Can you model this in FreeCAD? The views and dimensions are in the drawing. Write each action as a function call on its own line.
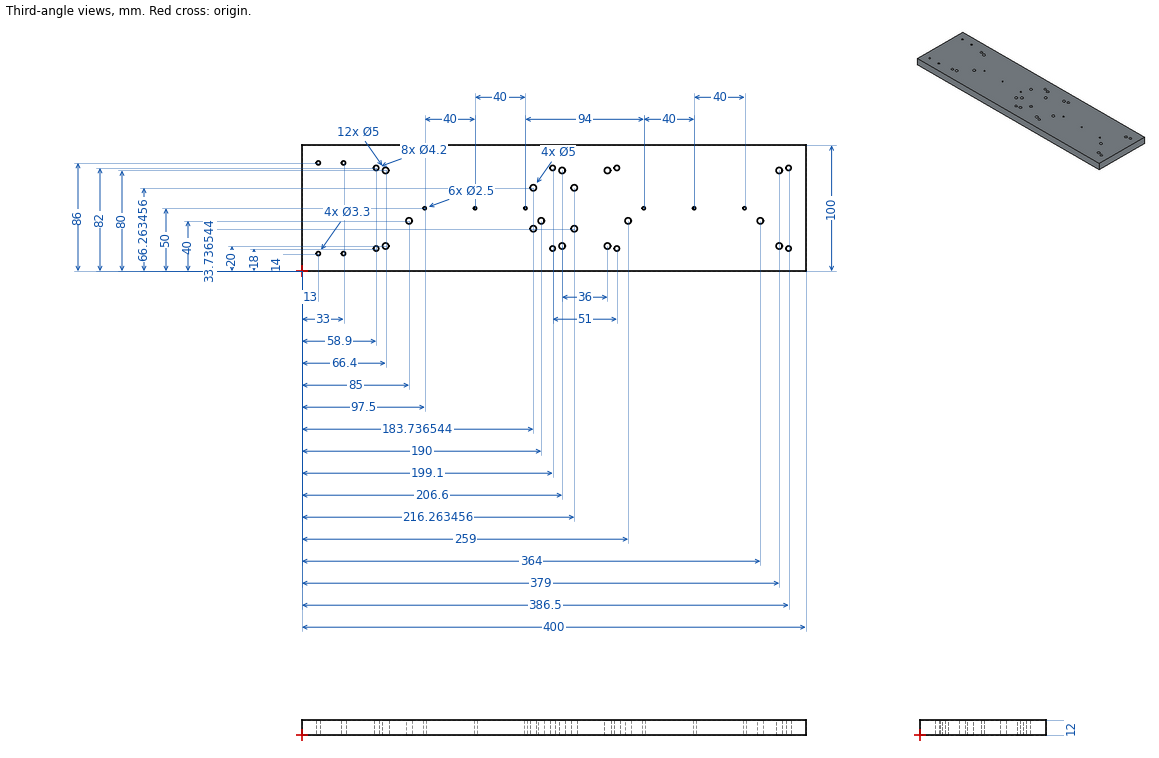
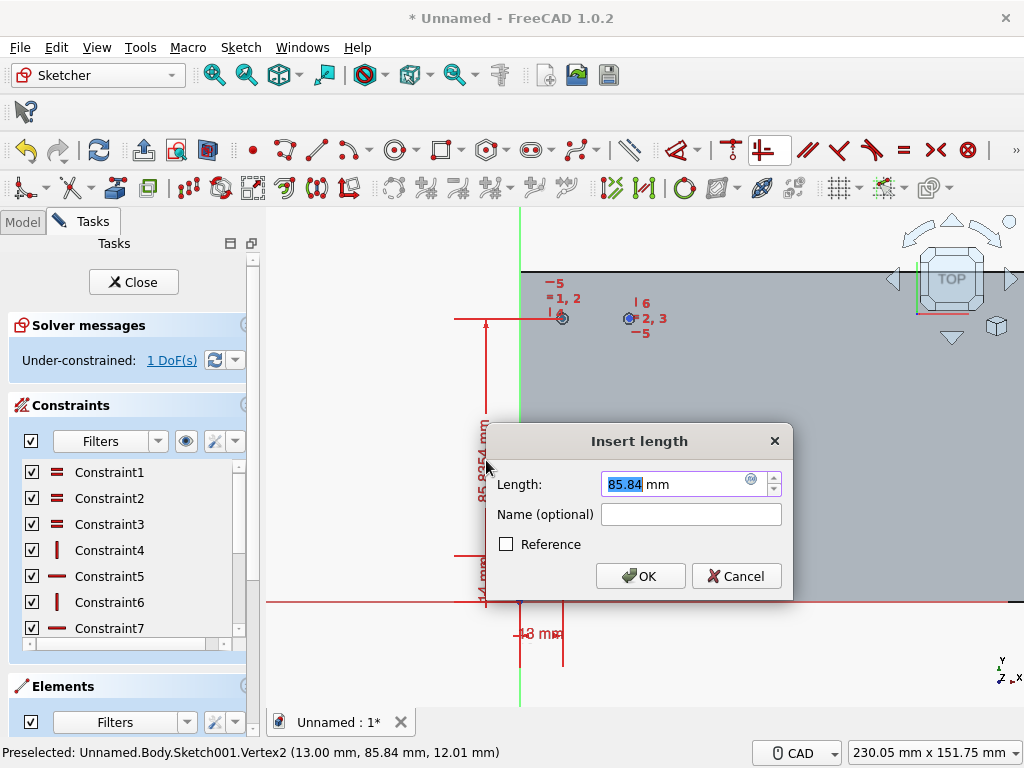
text(86)
key(Return)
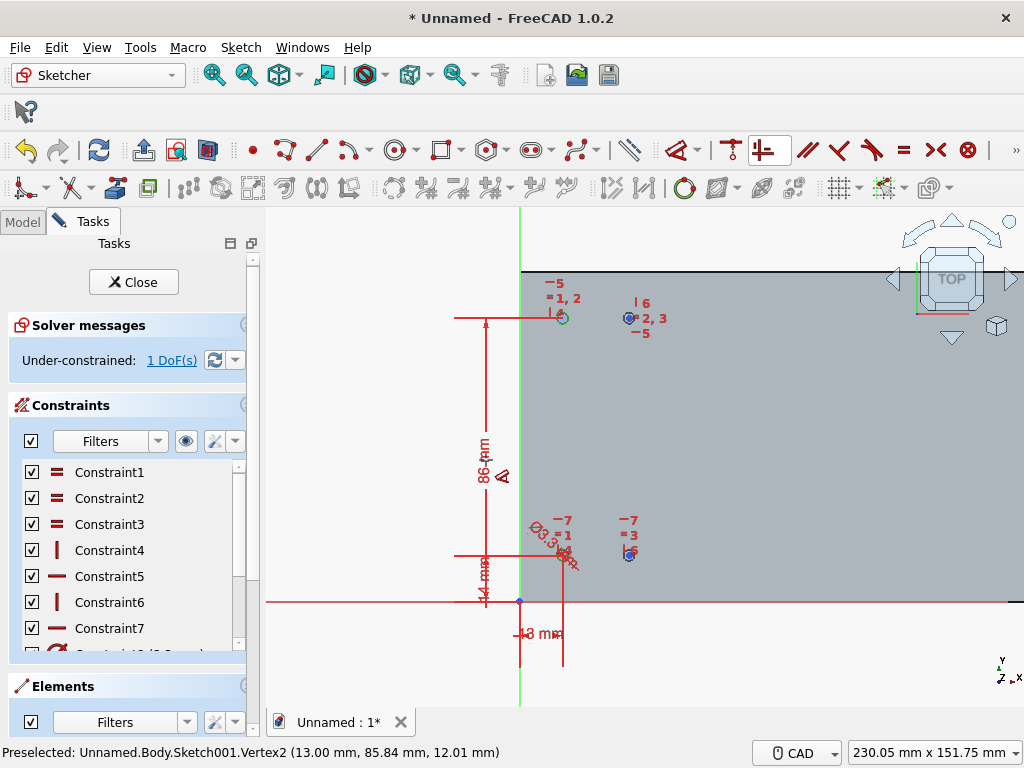
click(629, 318)
click(613, 636)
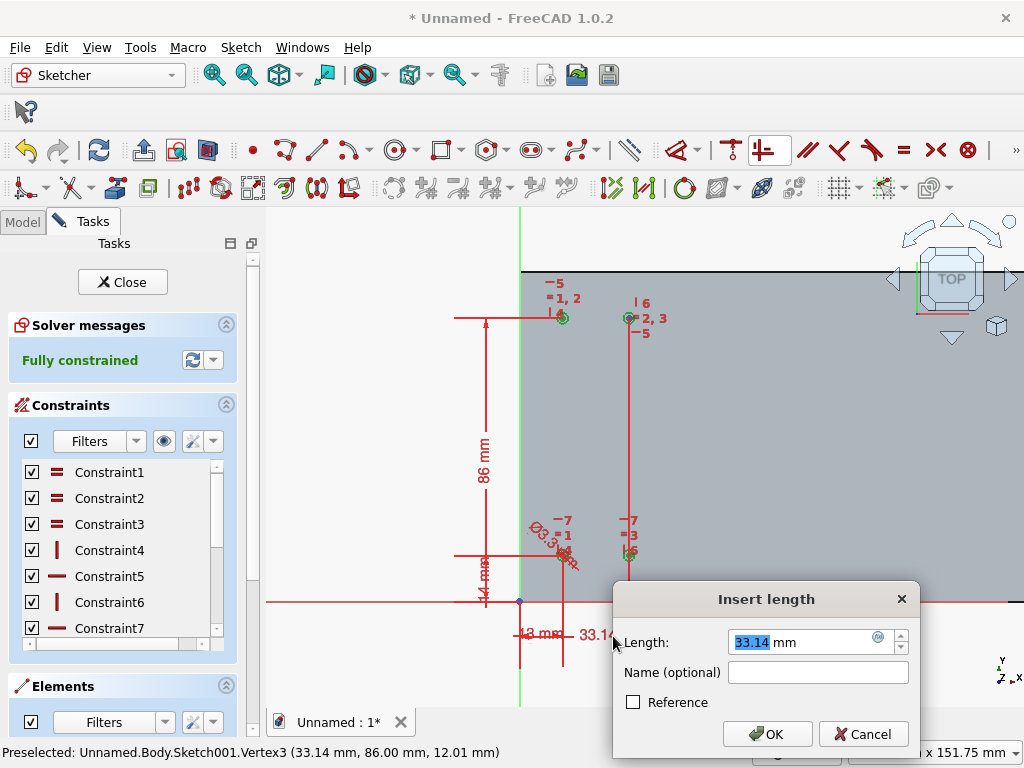
text(33)
key(Return)
key(Escape)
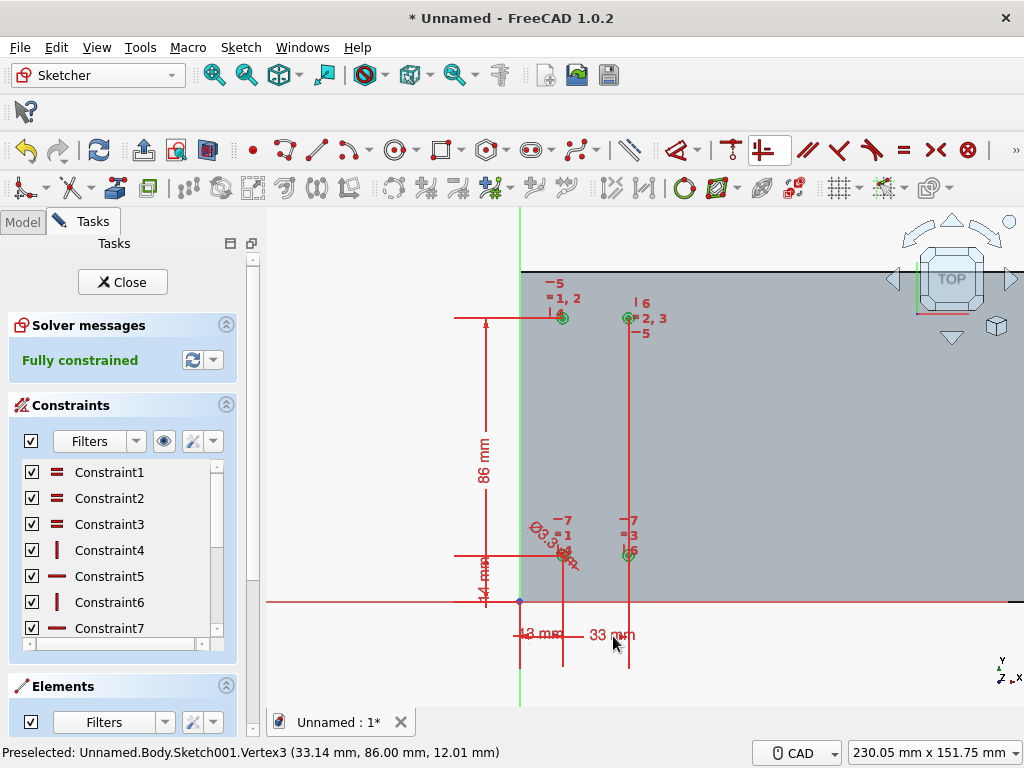
click(123, 282)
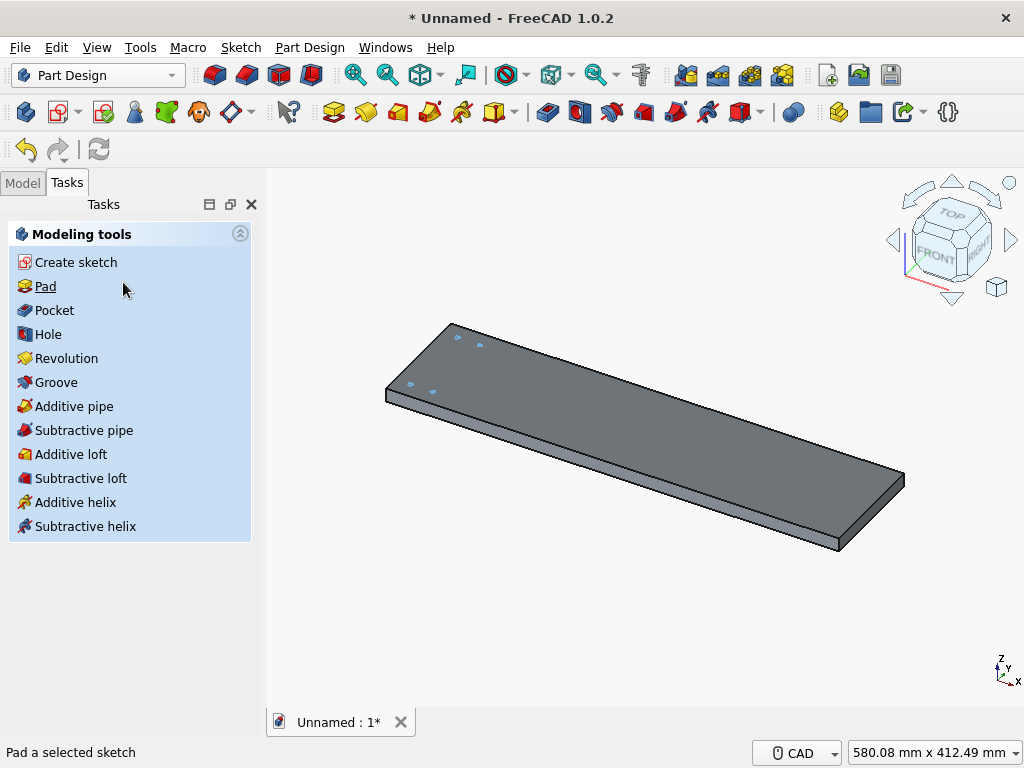
click(548, 112)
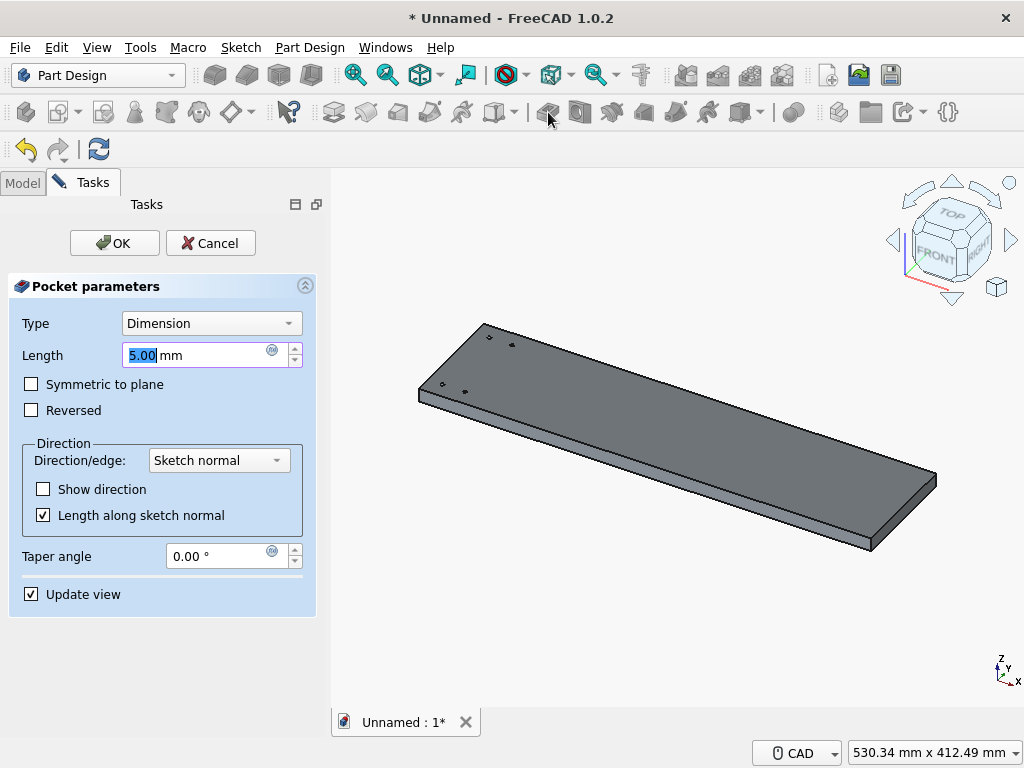
click(212, 324)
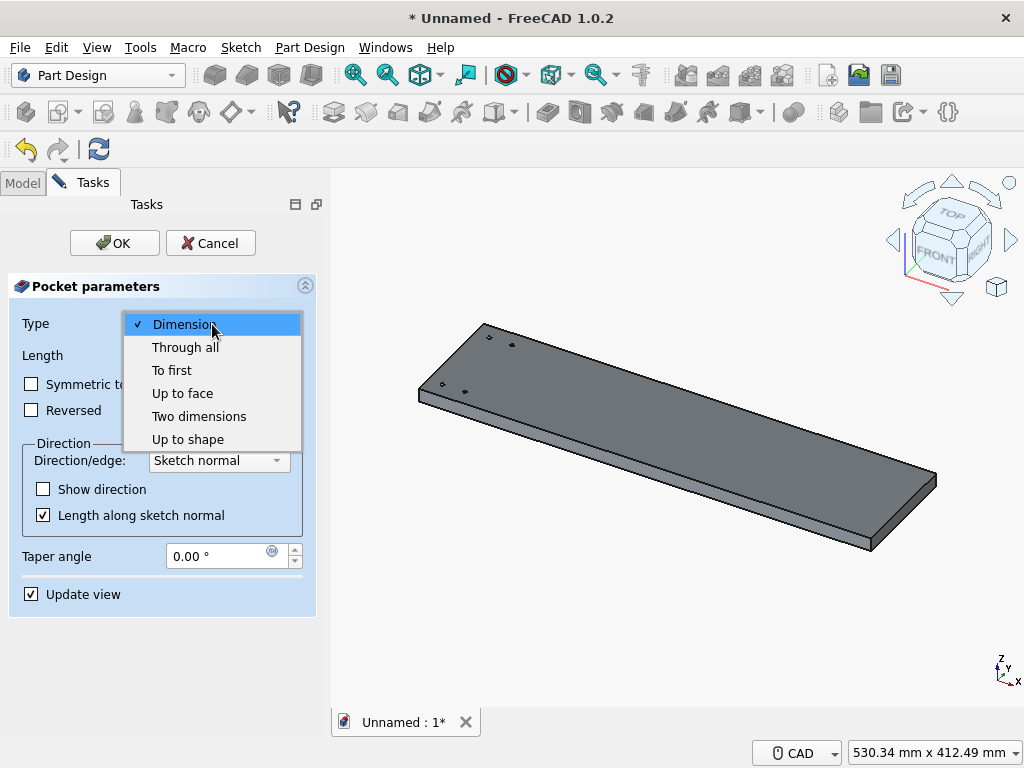
click(212, 348)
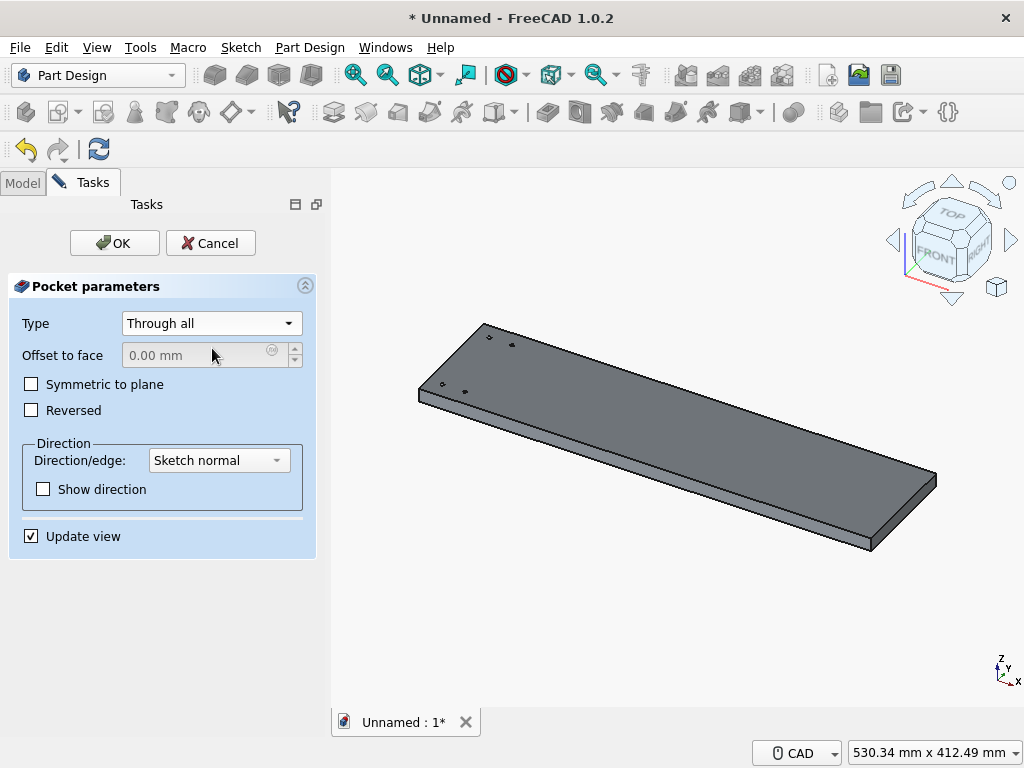
click(115, 243)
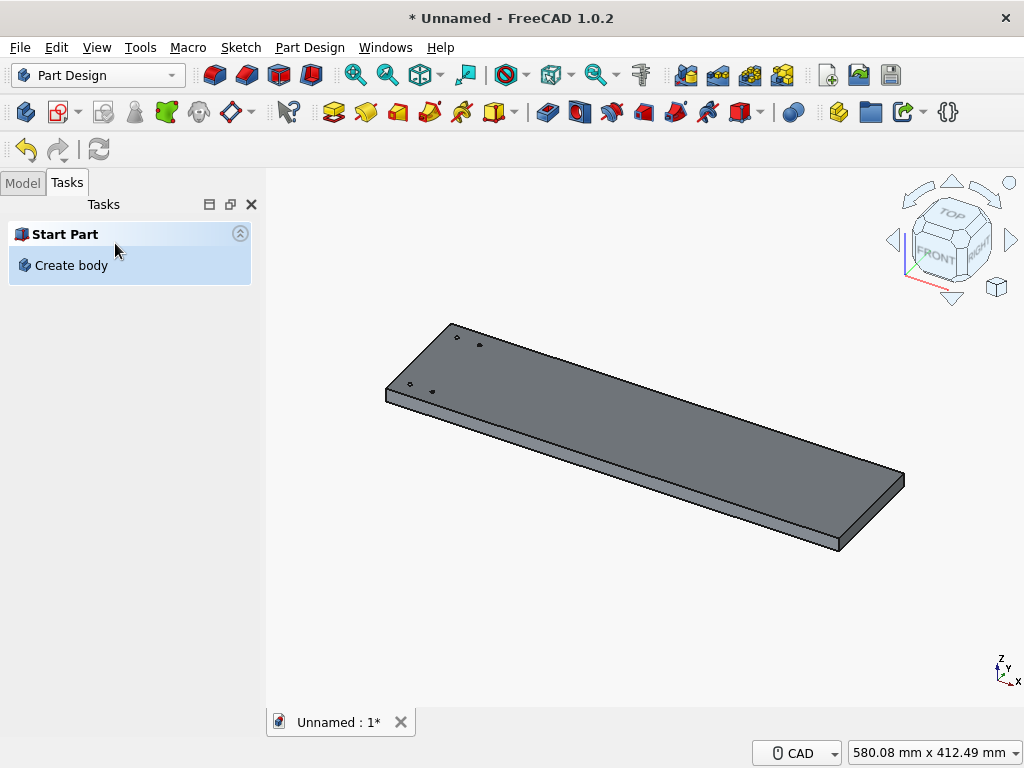
click(774, 473)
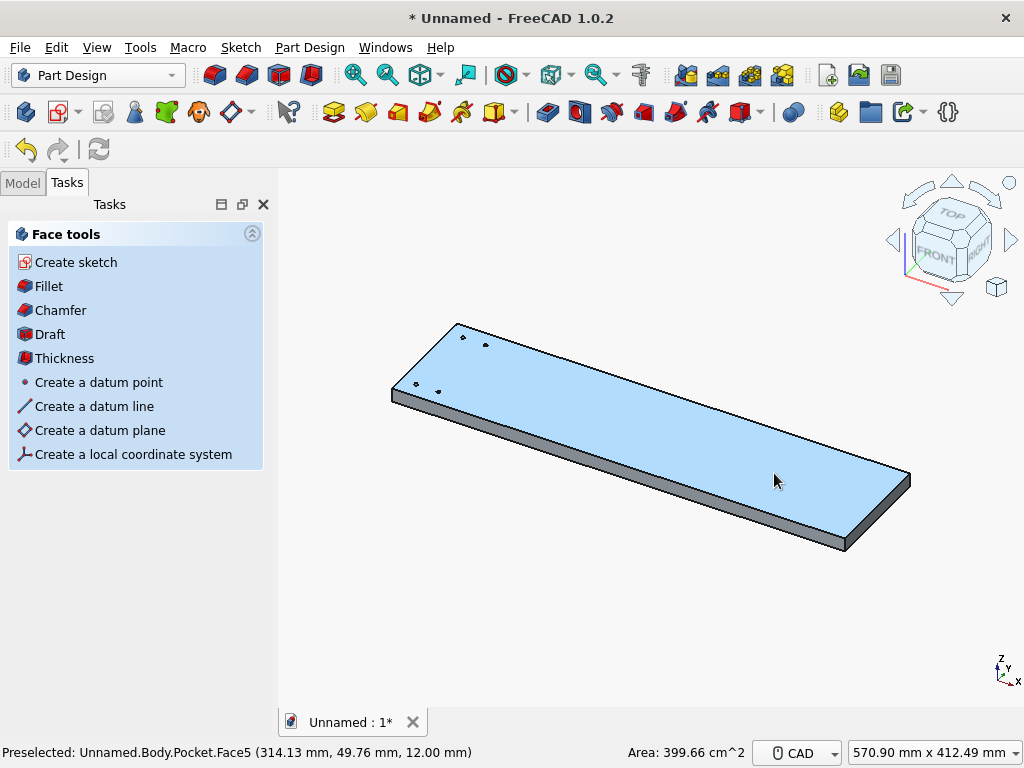
click(58, 112)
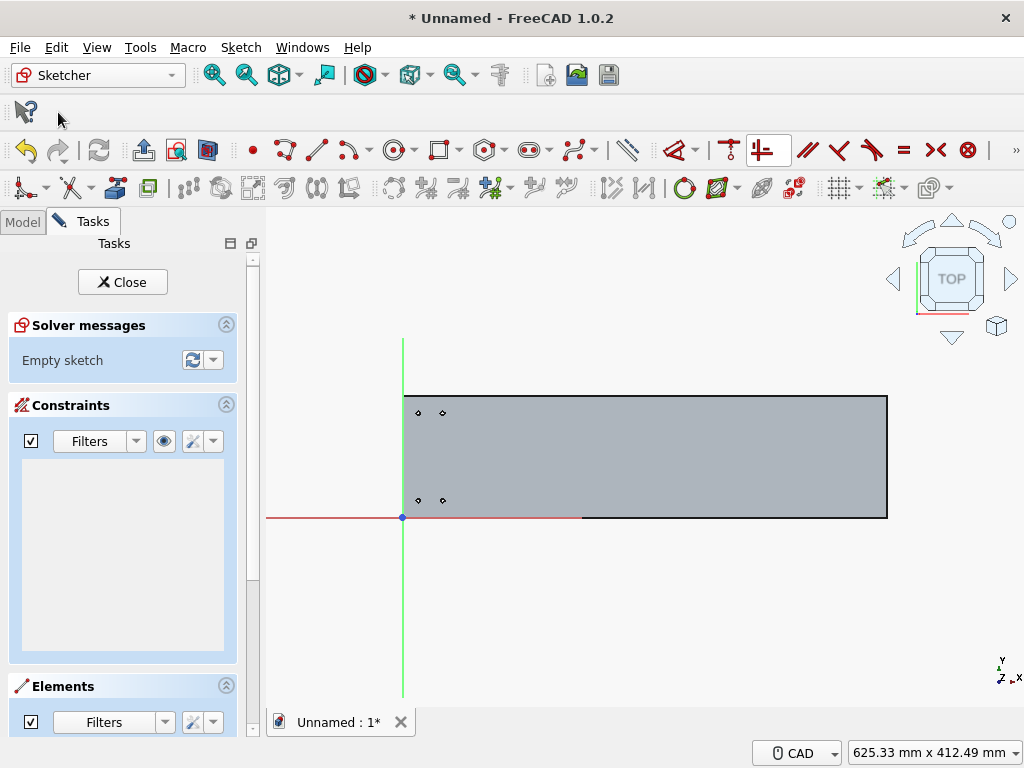
scroll(298, 413, down, 1)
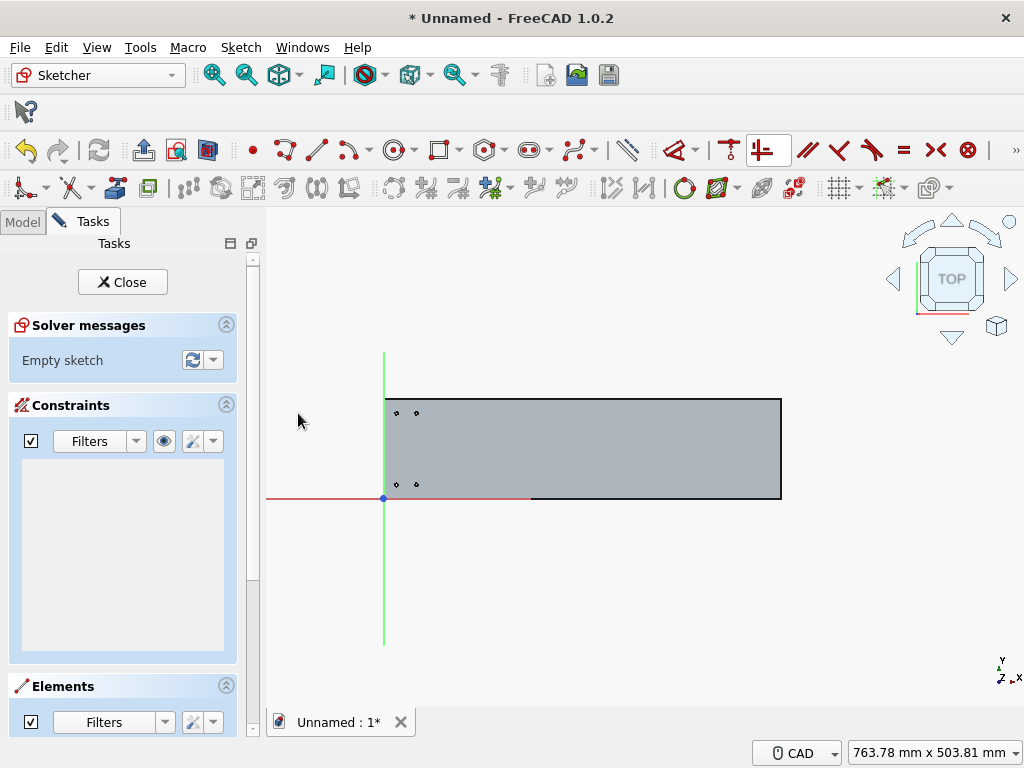
click(394, 150)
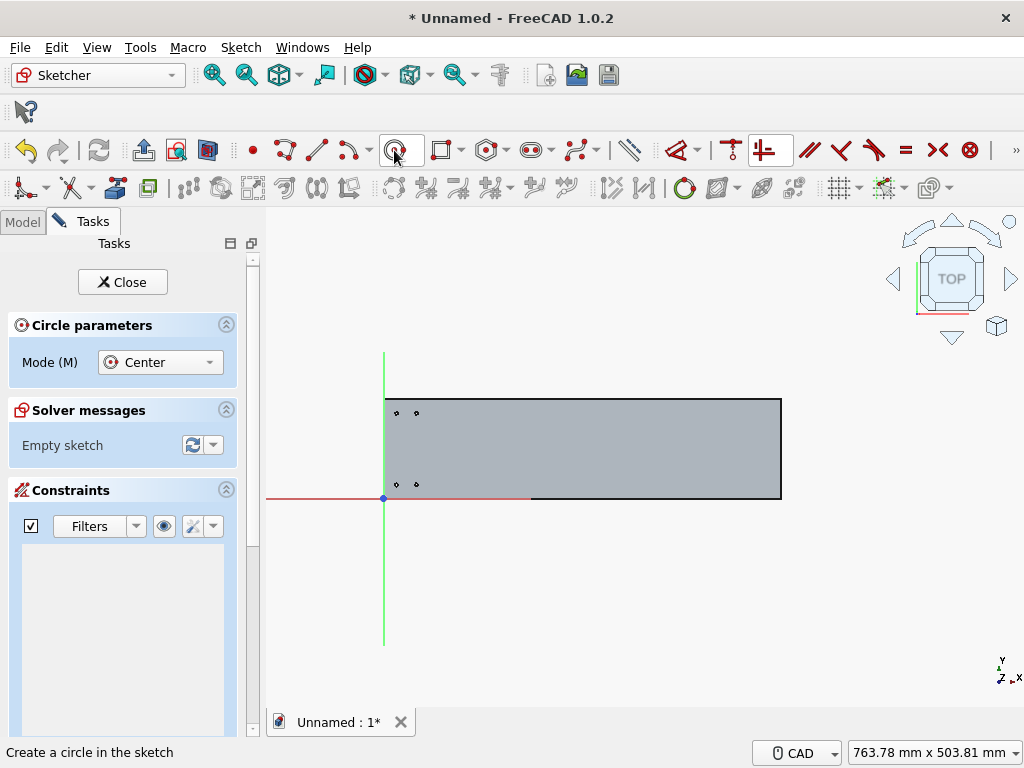
scroll(442, 417, up, 12)